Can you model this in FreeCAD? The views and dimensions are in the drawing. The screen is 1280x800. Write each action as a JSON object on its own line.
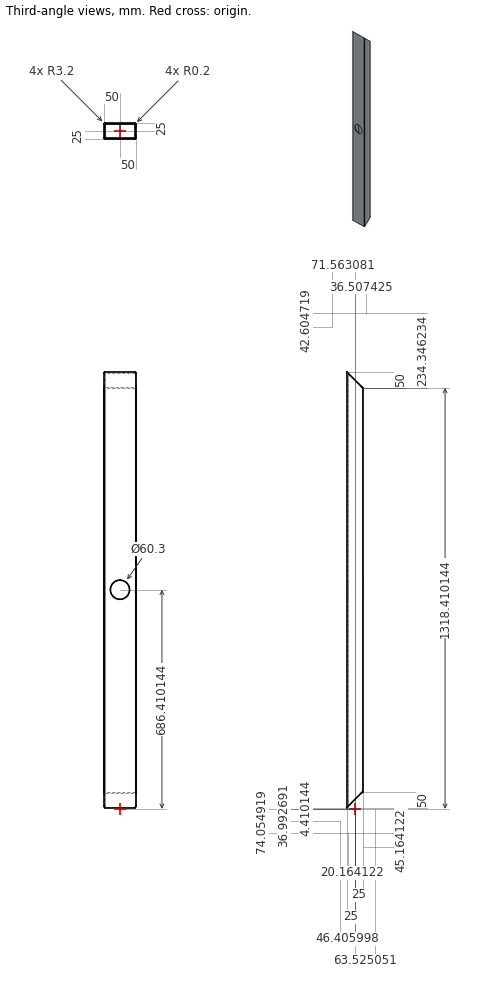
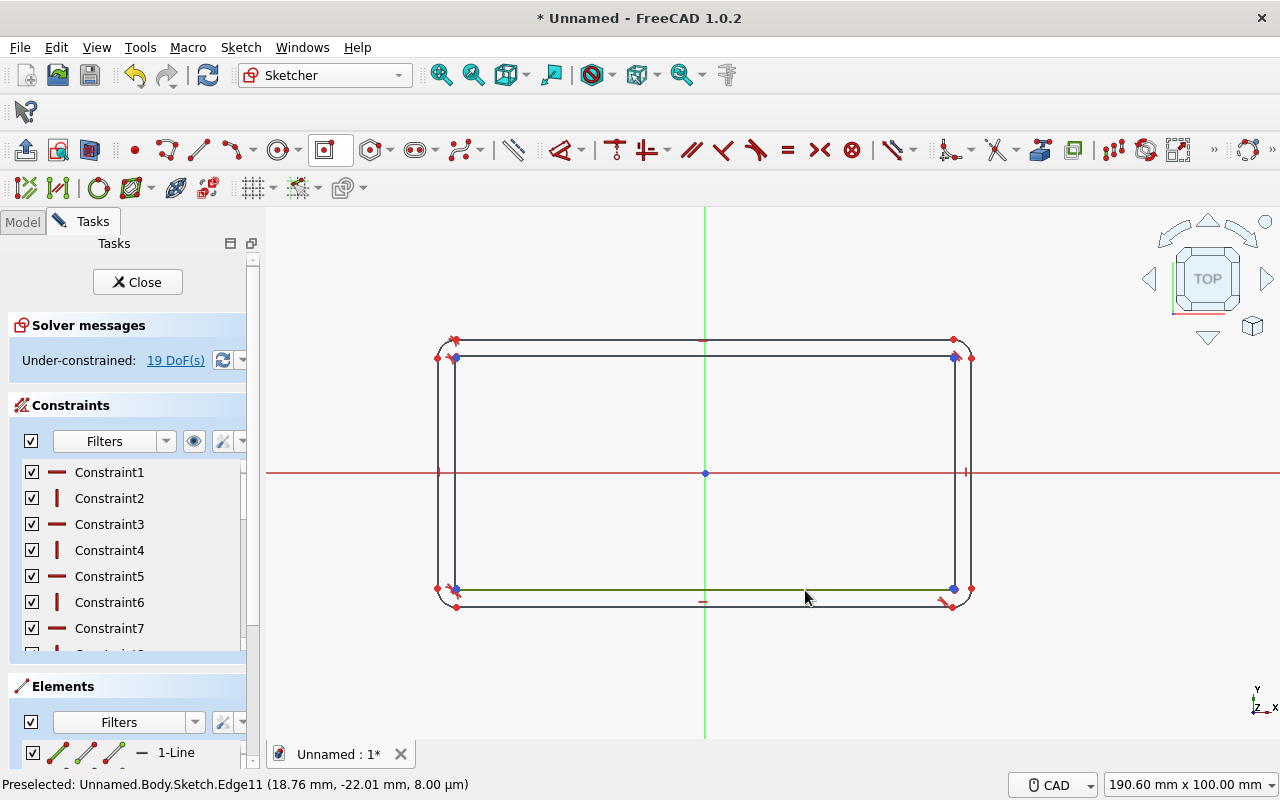
{"action": "scroll", "coordinate": [455, 590], "scroll_direction": "up", "scroll_amount": 14}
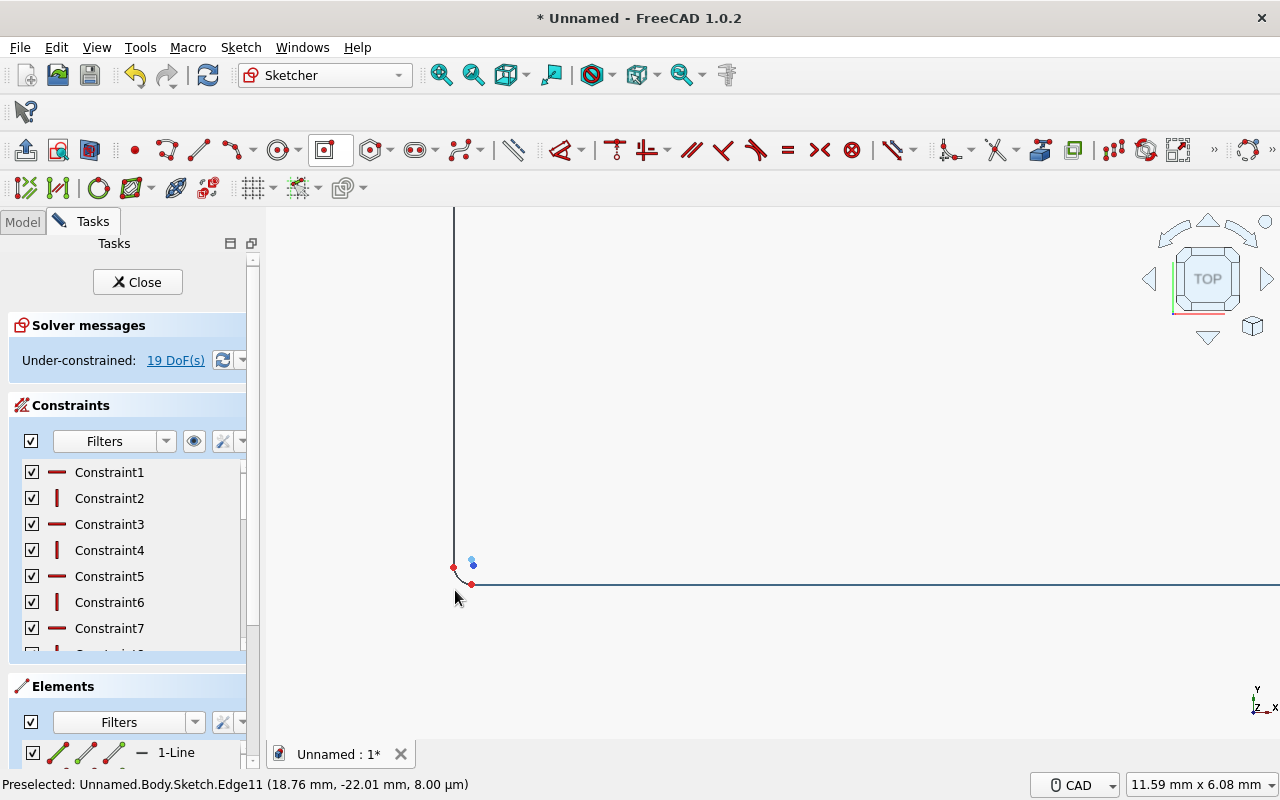
{"action": "left_click", "coordinate": [460, 579]}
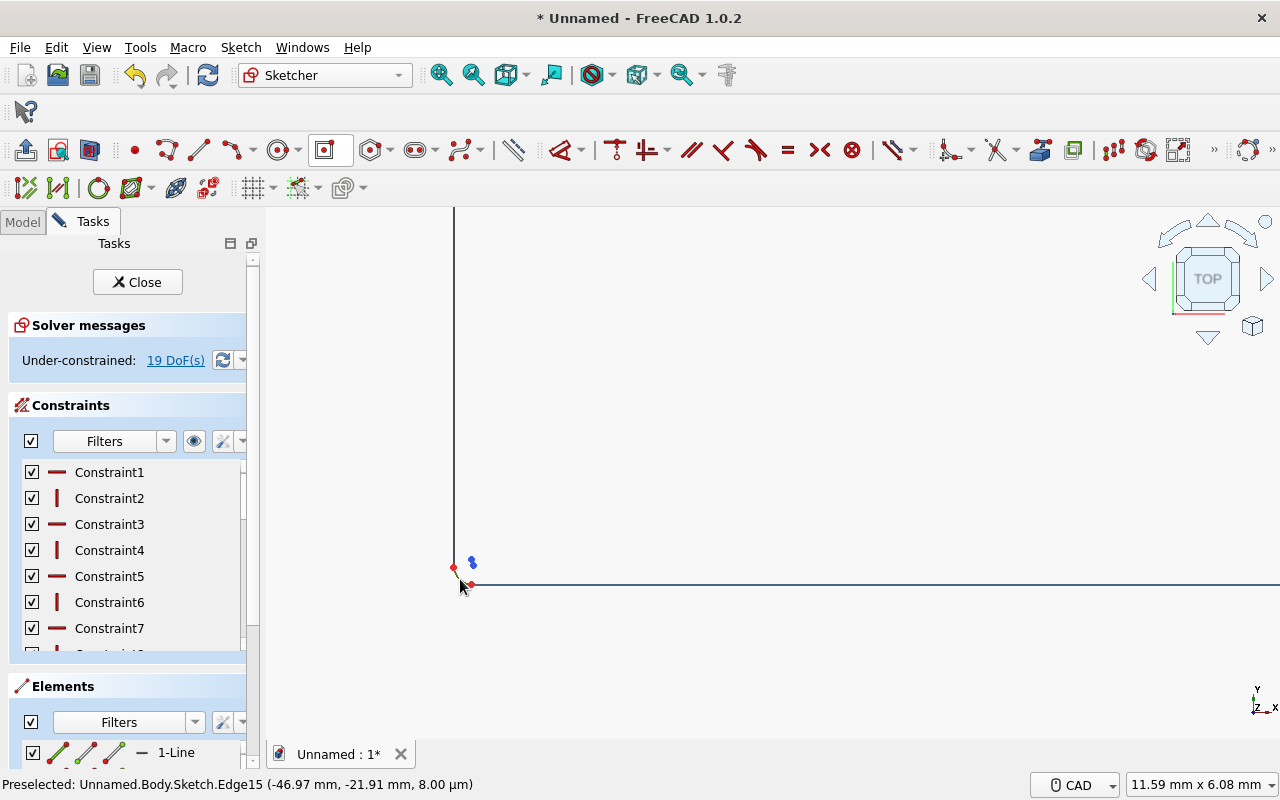
{"action": "left_click", "coordinate": [756, 150]}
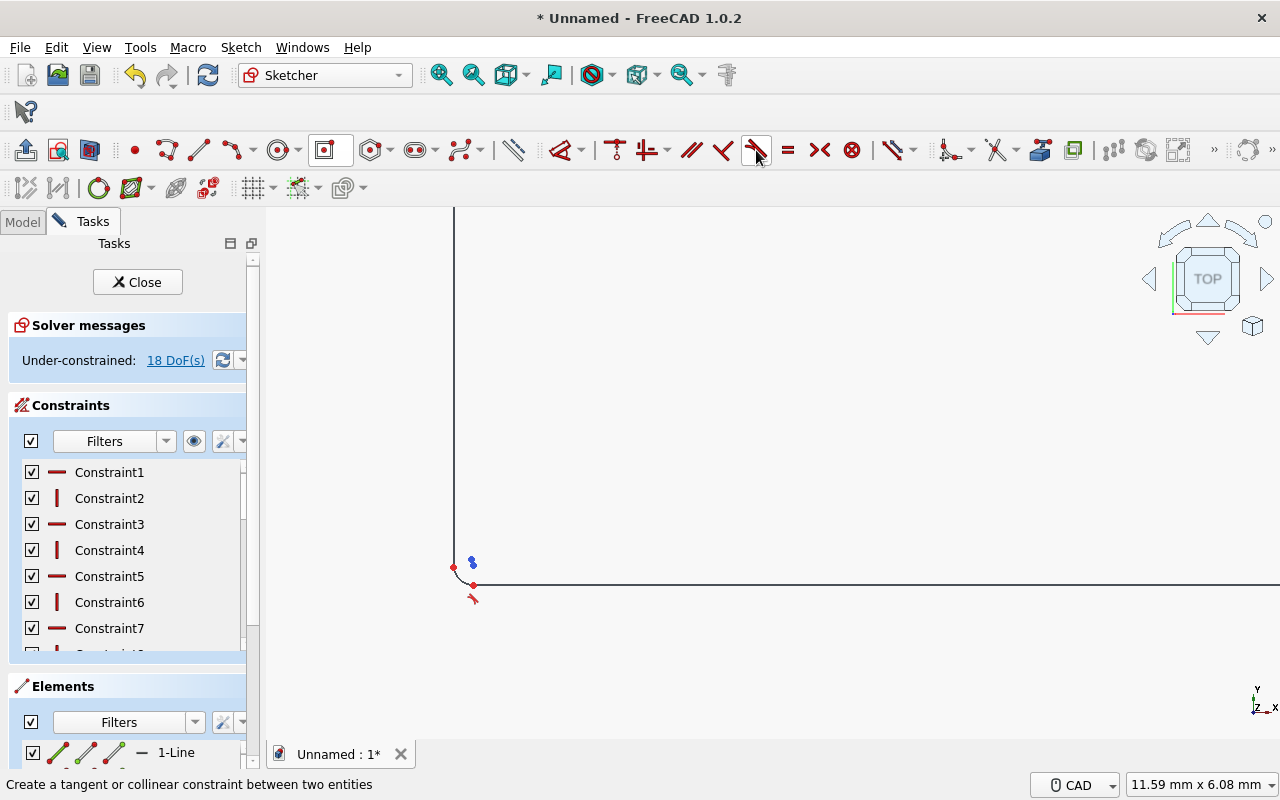
{"action": "scroll", "coordinate": [454, 590], "scroll_direction": "down", "scroll_amount": 14}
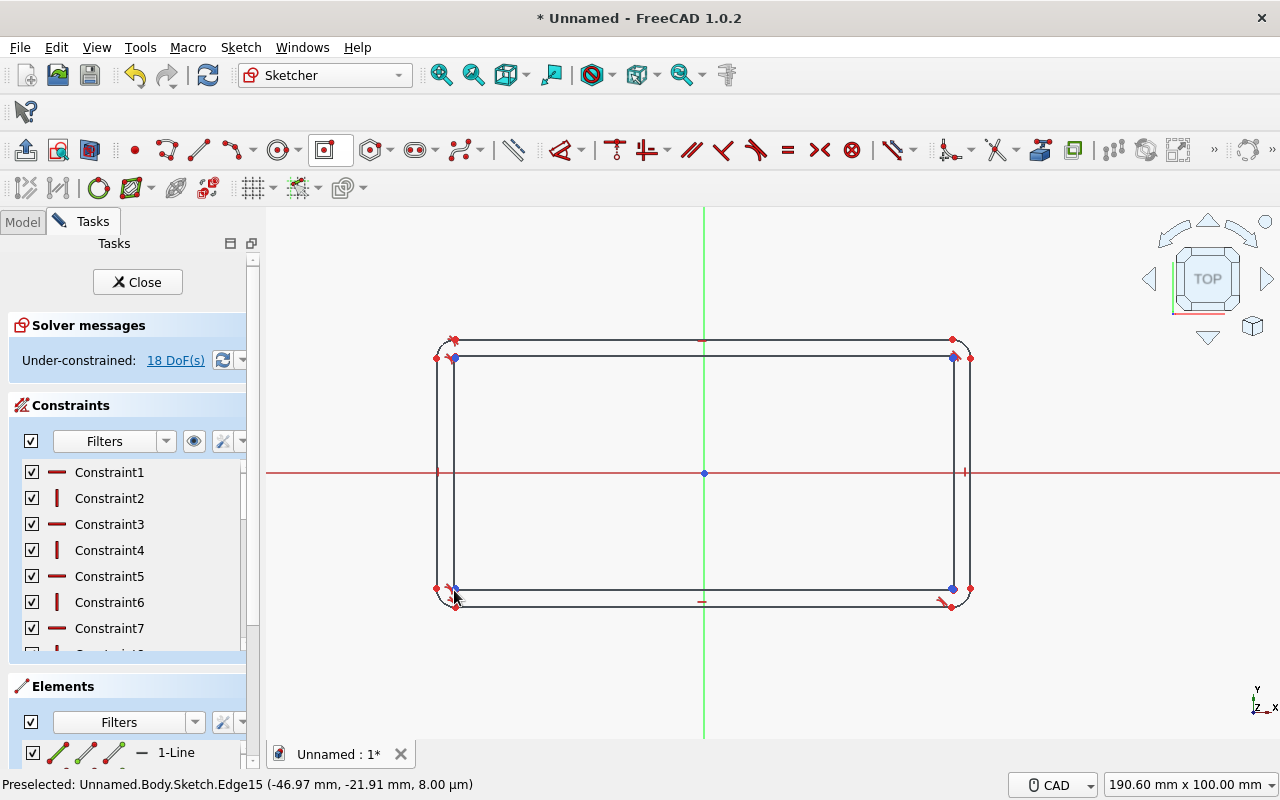
{"action": "left_click", "coordinate": [454, 520]}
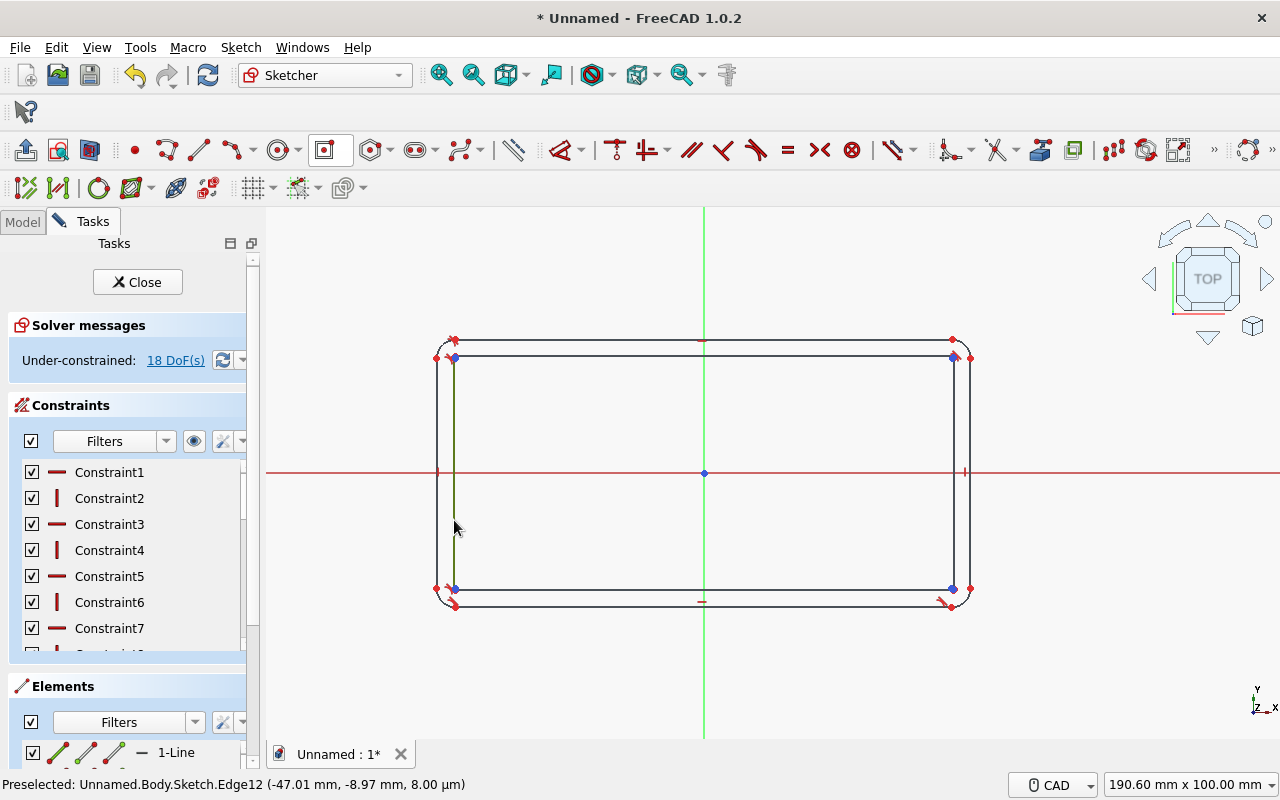
{"action": "scroll", "coordinate": [455, 590], "scroll_direction": "up", "scroll_amount": 14}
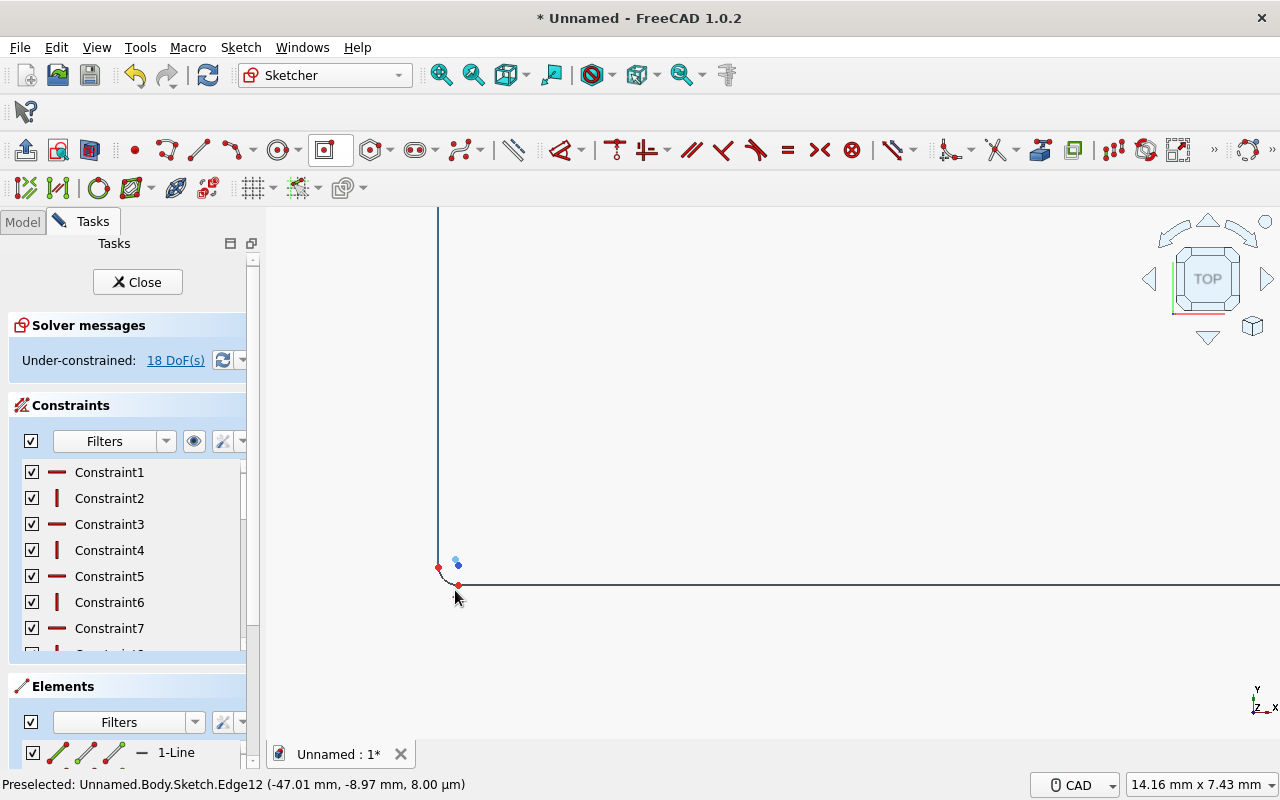
{"action": "left_click", "coordinate": [445, 580]}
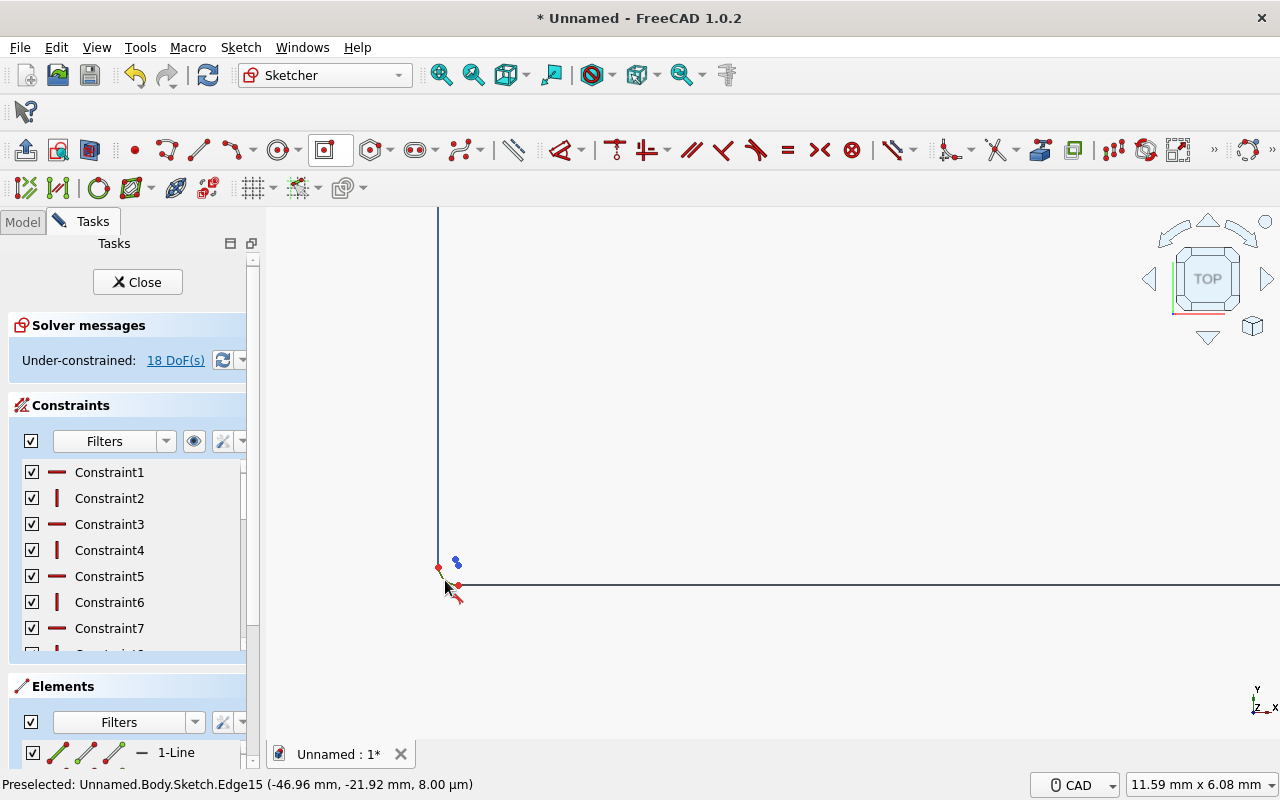
{"action": "left_click", "coordinate": [756, 150]}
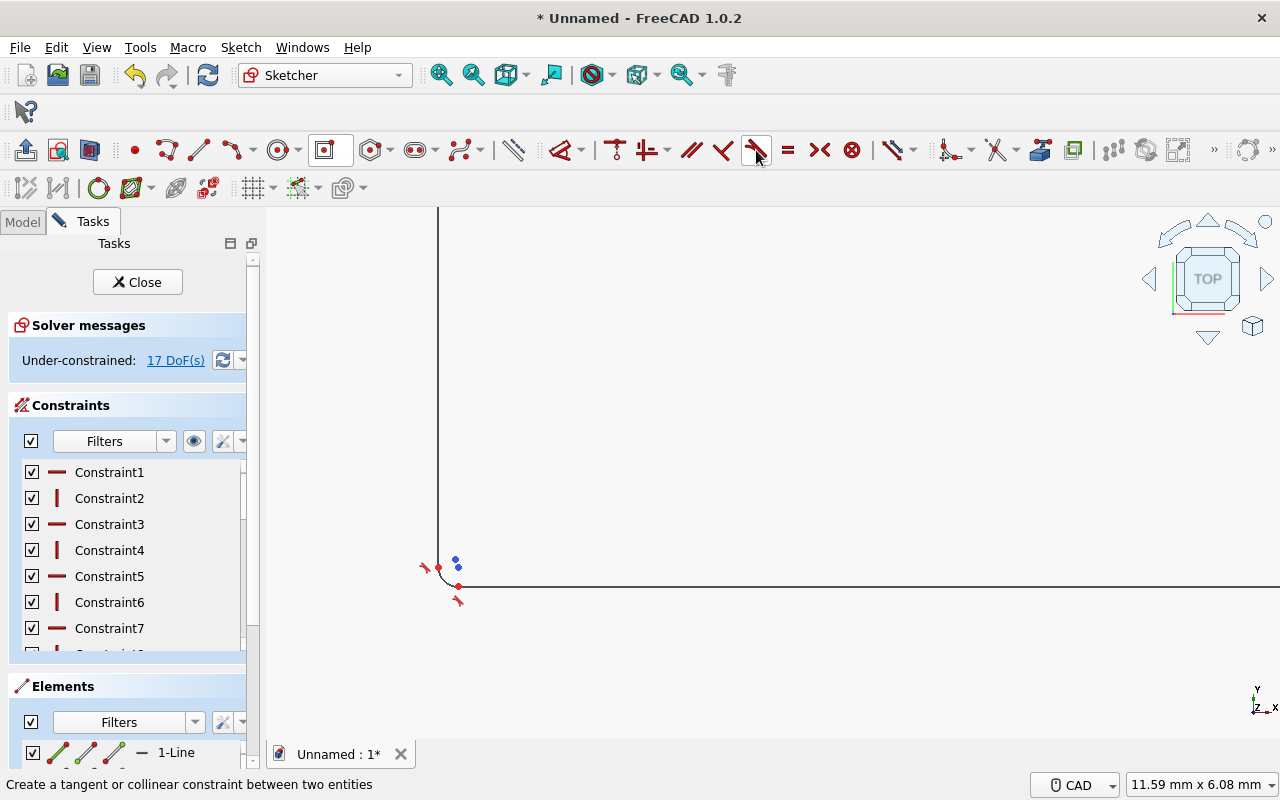
{"action": "scroll", "coordinate": [455, 590], "scroll_direction": "down", "scroll_amount": 14}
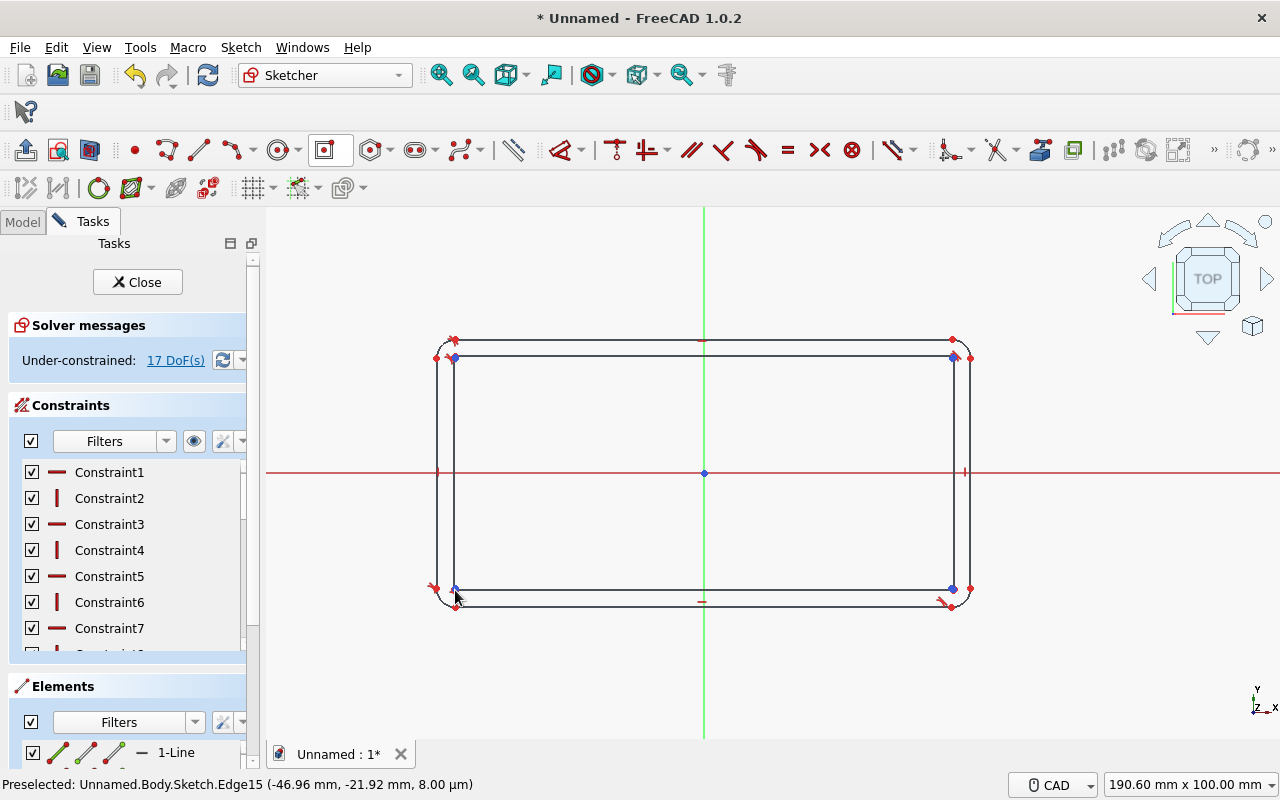
{"action": "left_click", "coordinate": [454, 520]}